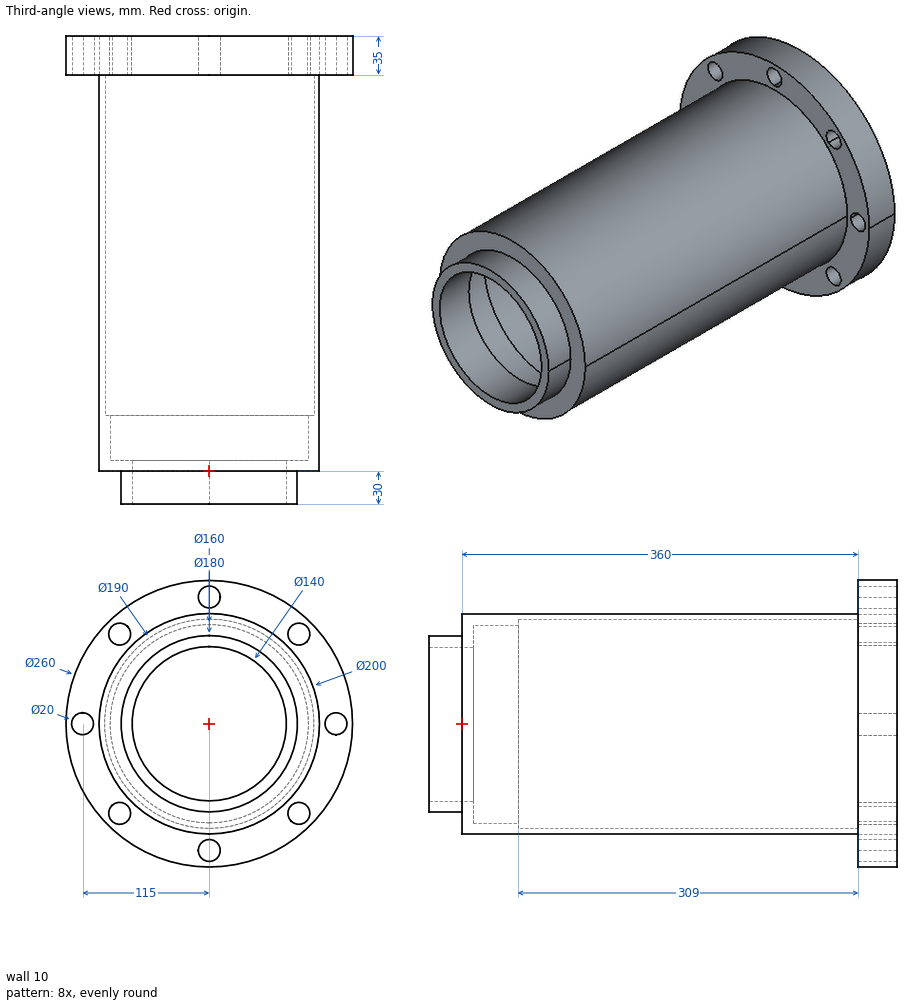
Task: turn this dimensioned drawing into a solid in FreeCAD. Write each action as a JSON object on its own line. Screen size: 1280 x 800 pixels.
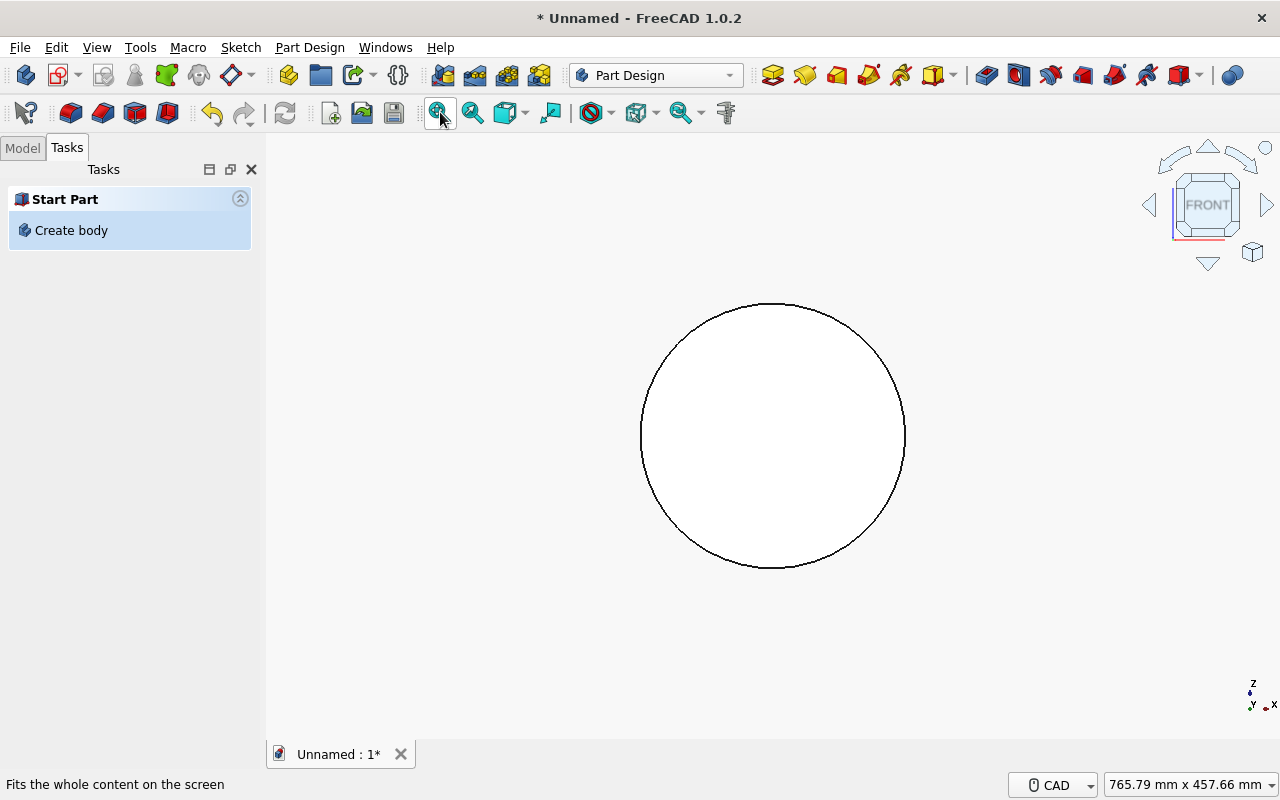
{"action": "key", "text": "3"}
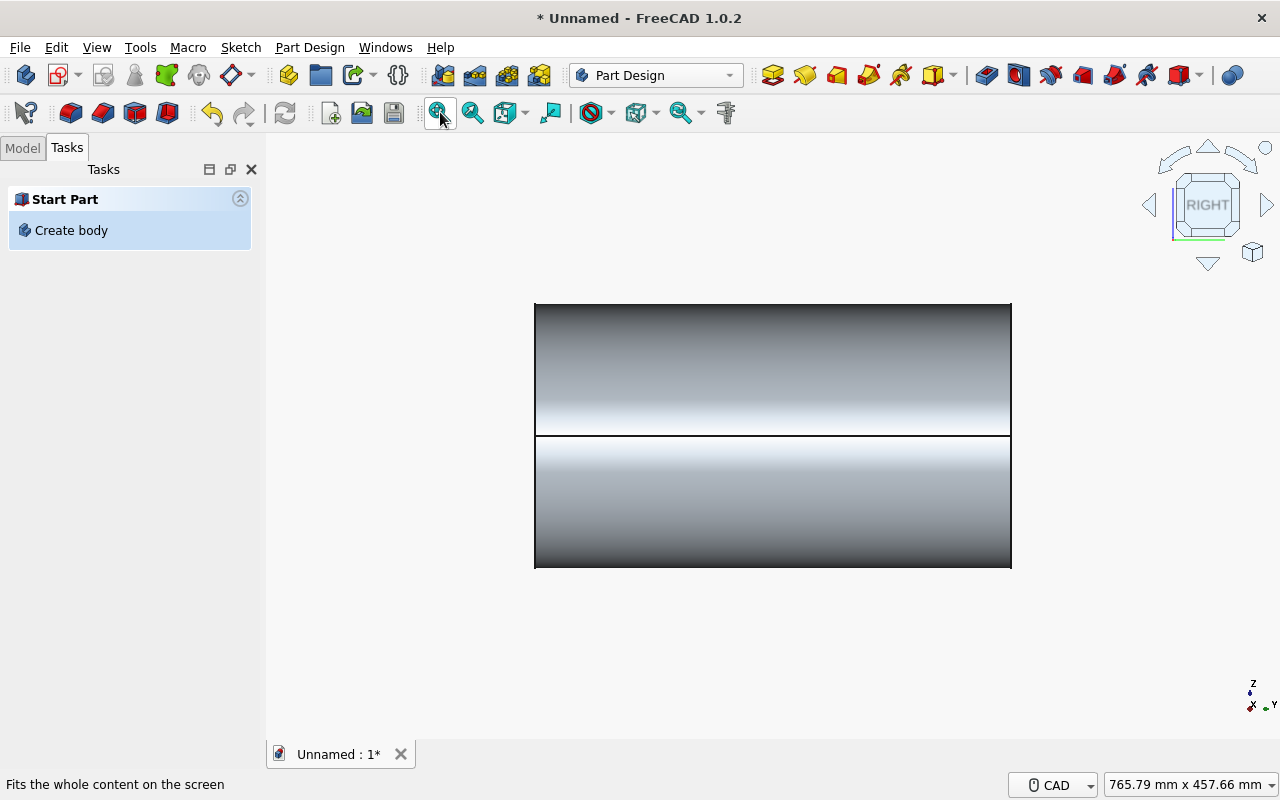
{"action": "key", "text": "5"}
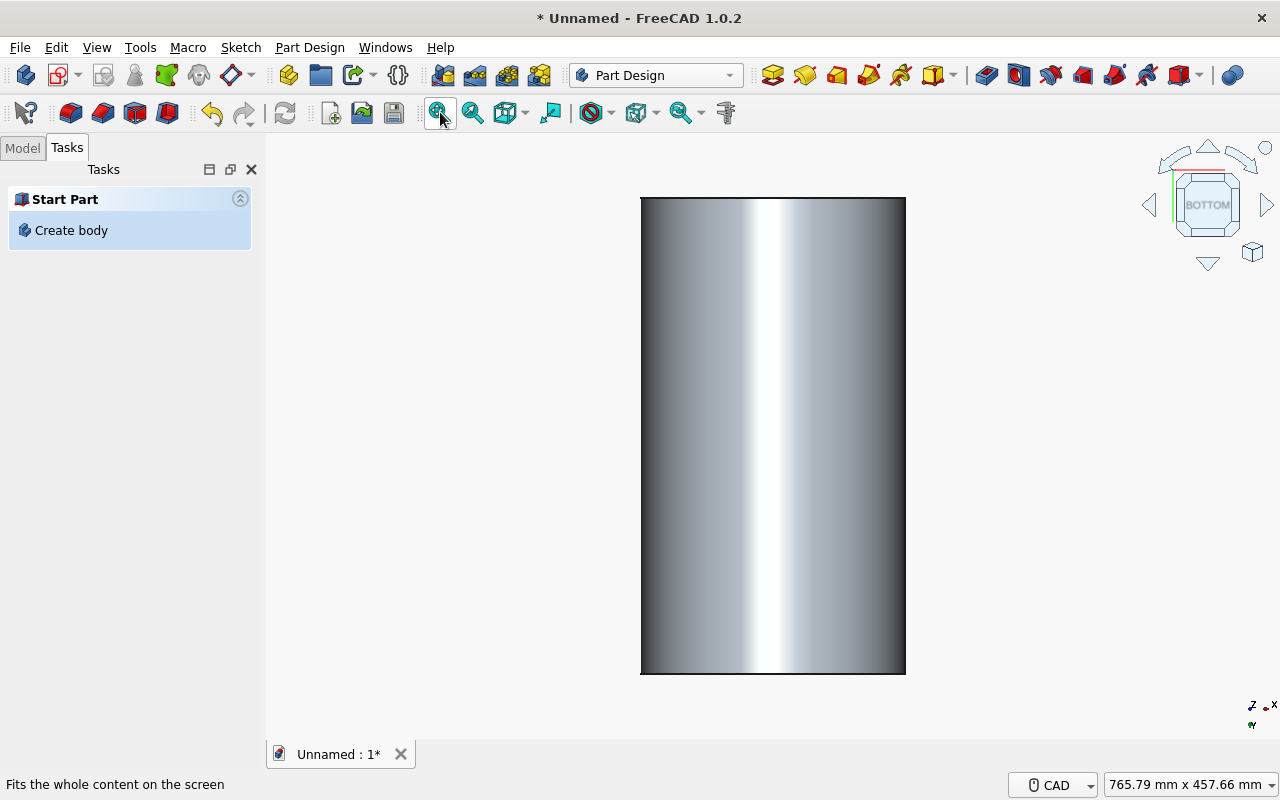
{"action": "key", "text": "4"}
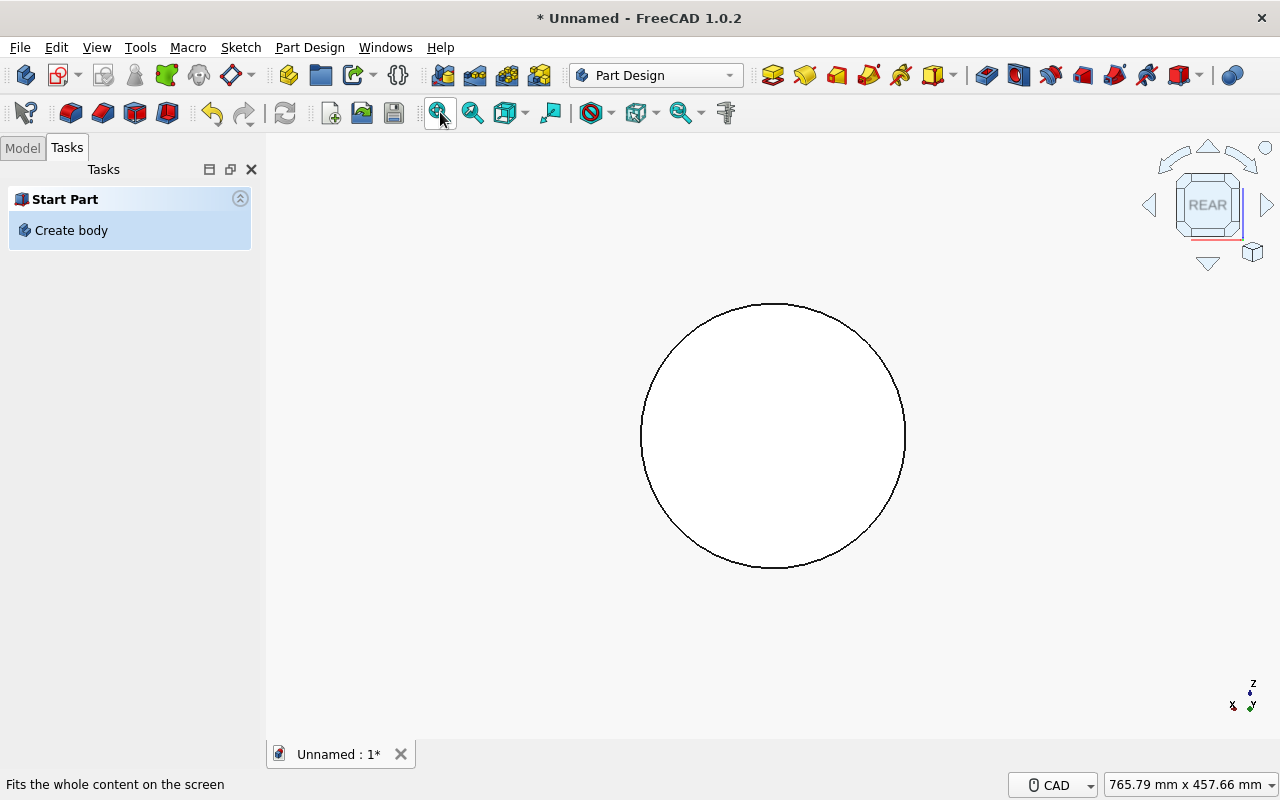
{"action": "key", "text": "v f"}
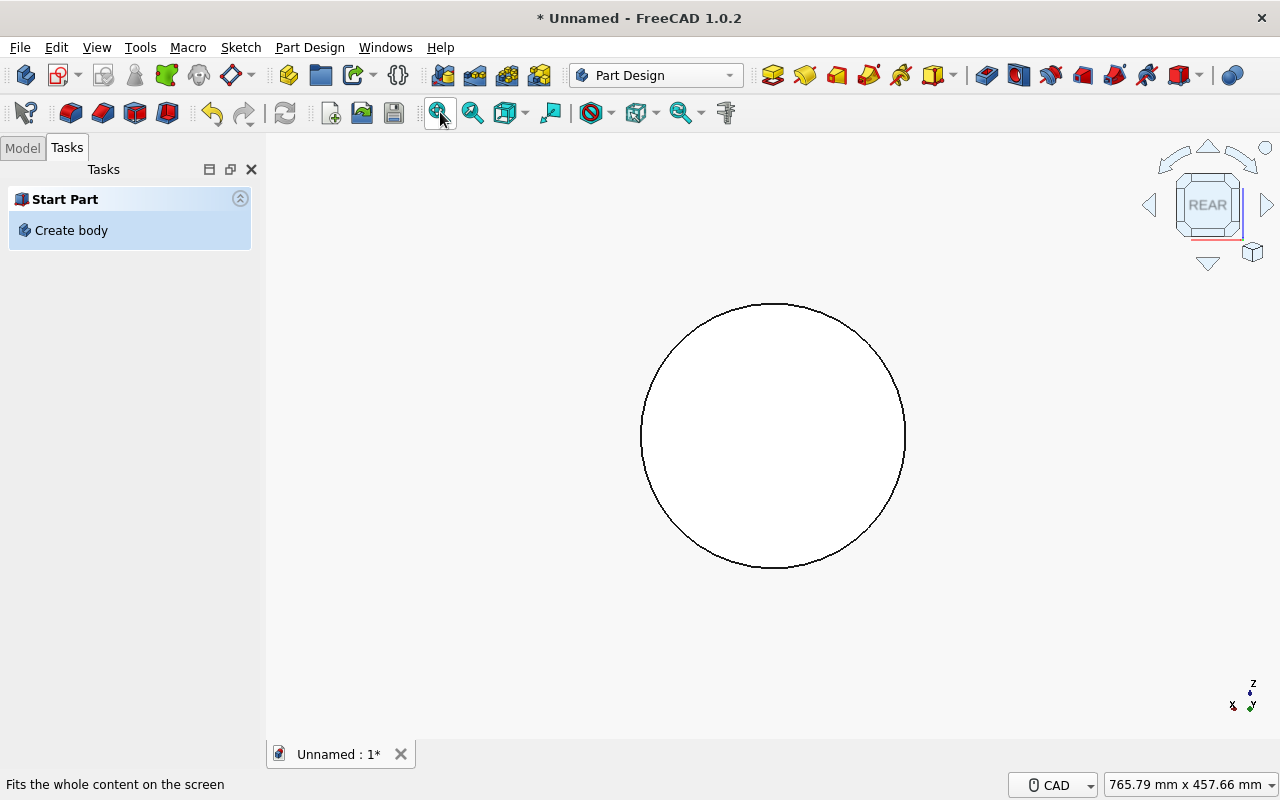
{"action": "left_click", "coordinate": [773, 435]}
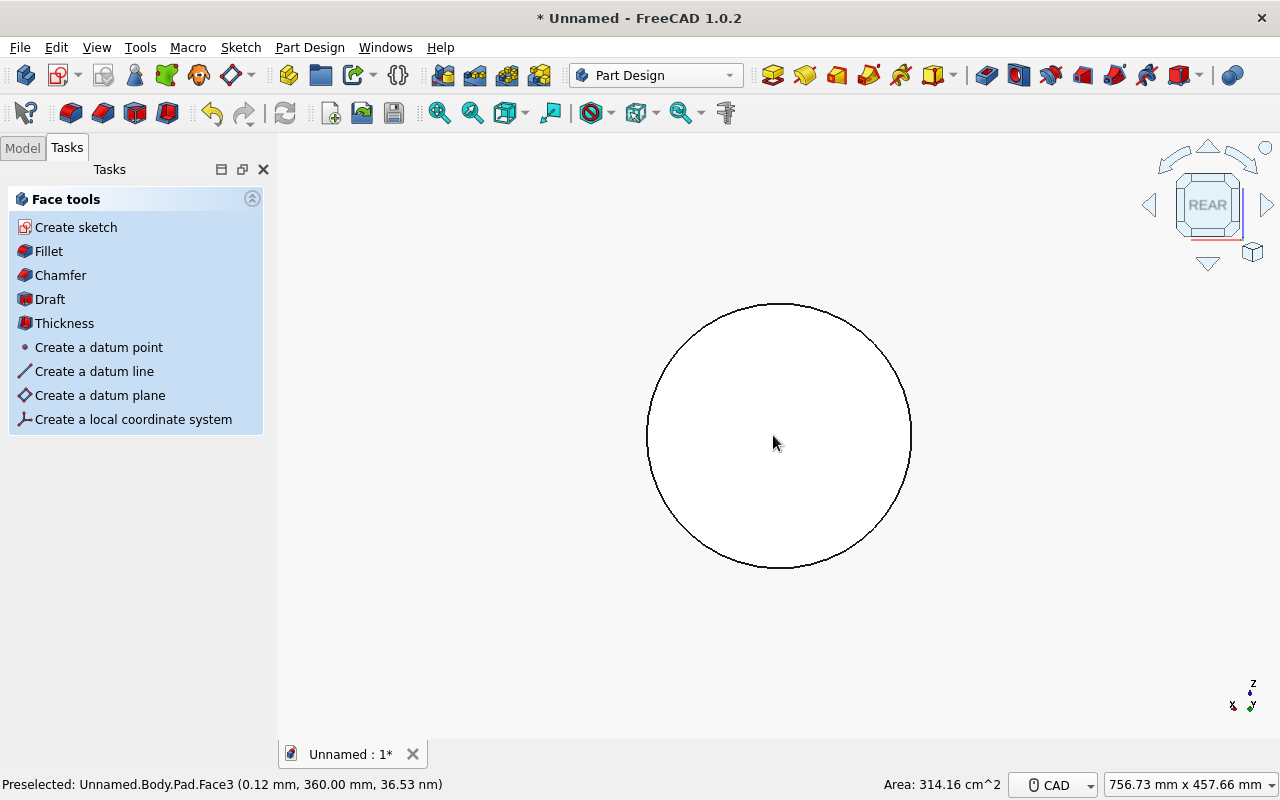
{"action": "left_click", "coordinate": [168, 114]}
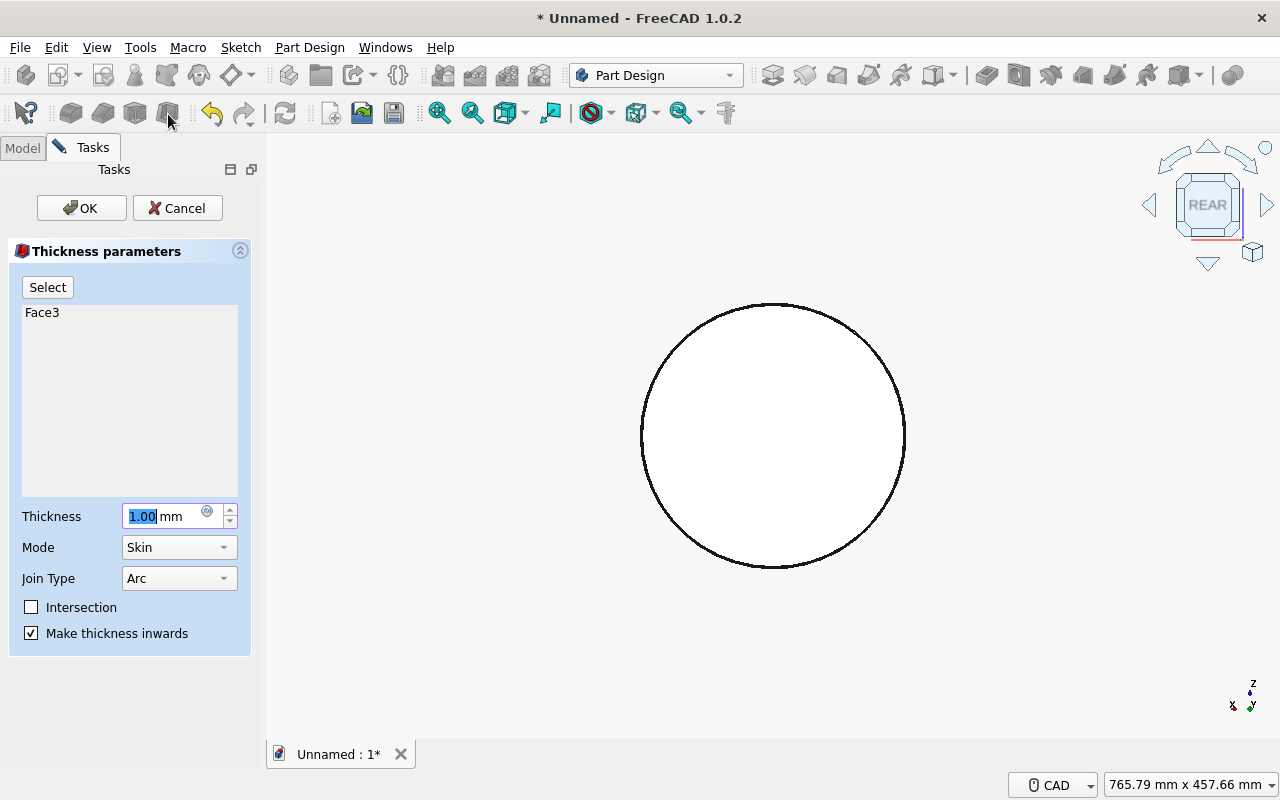
{"action": "type", "text": "10"}
{"action": "key", "text": "Tab"}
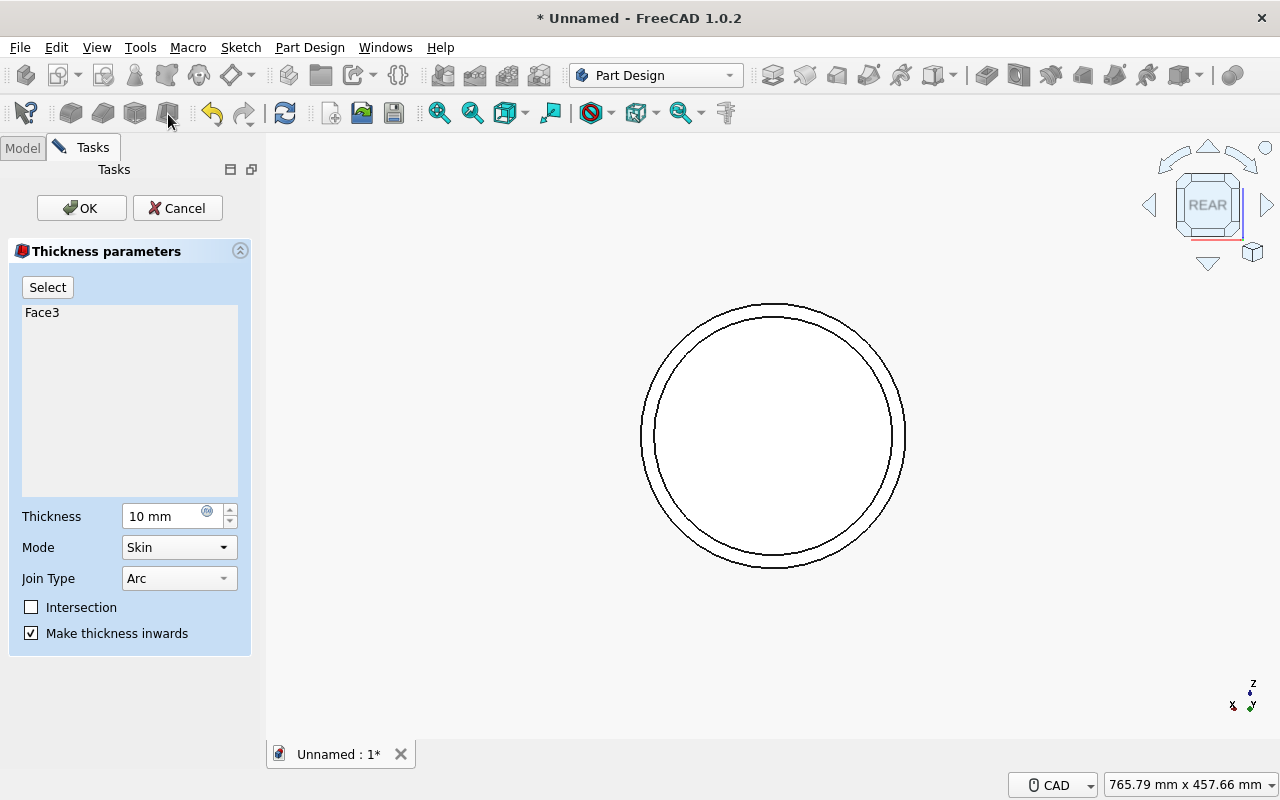
{"action": "left_click", "coordinate": [180, 578]}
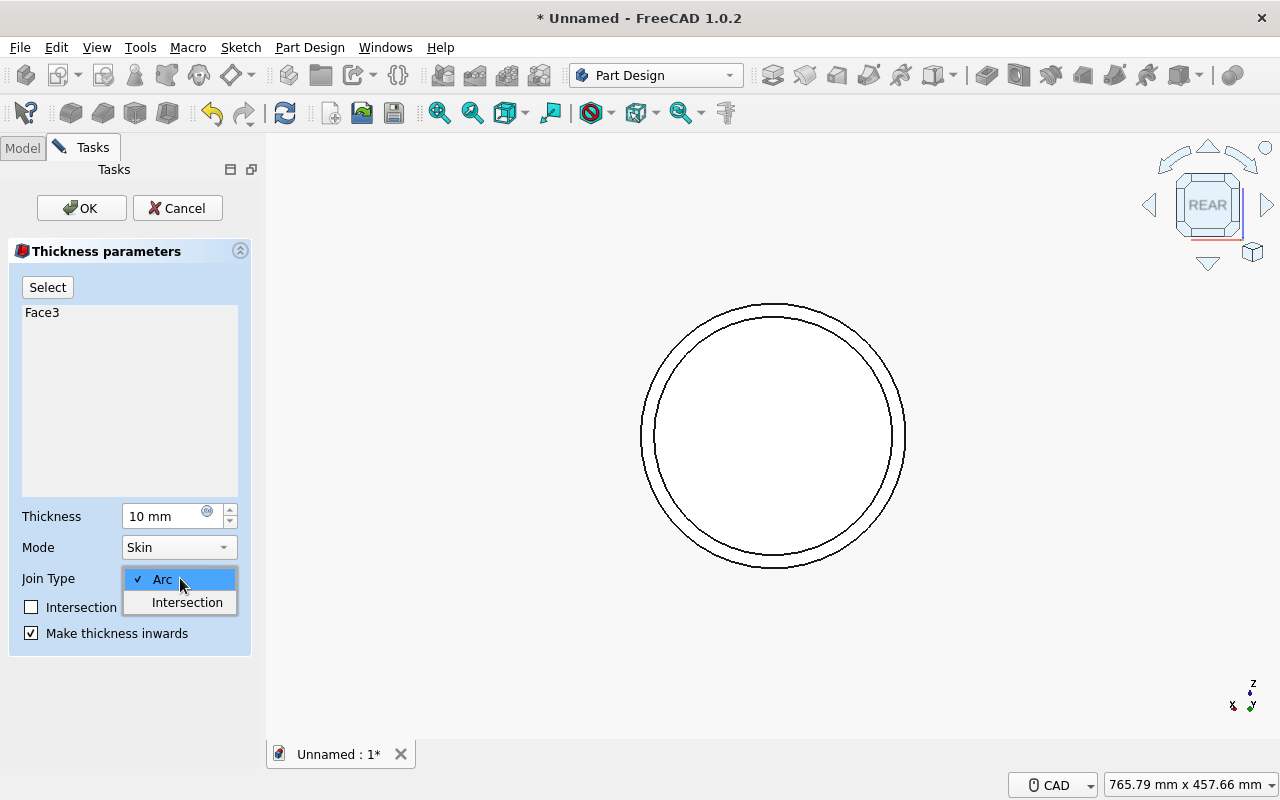
{"action": "left_click", "coordinate": [179, 602]}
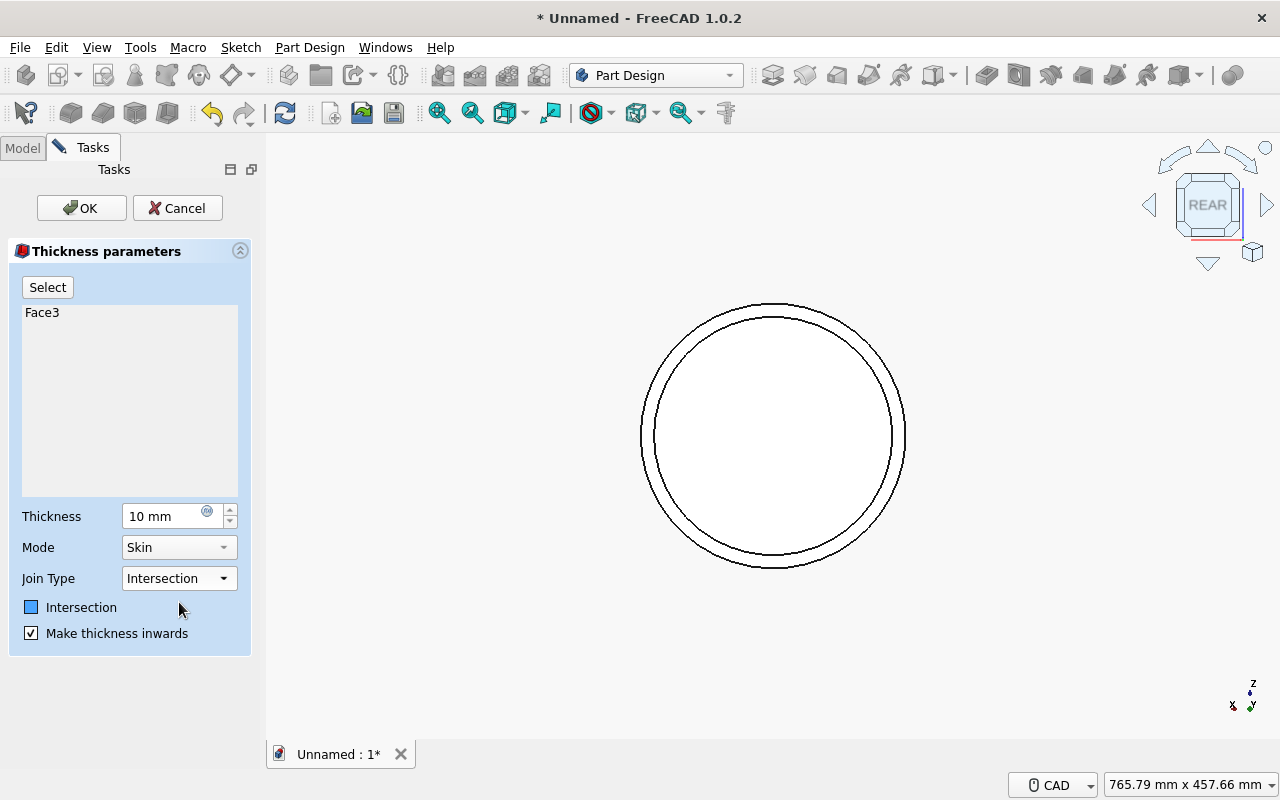
{"action": "left_click", "coordinate": [82, 208]}